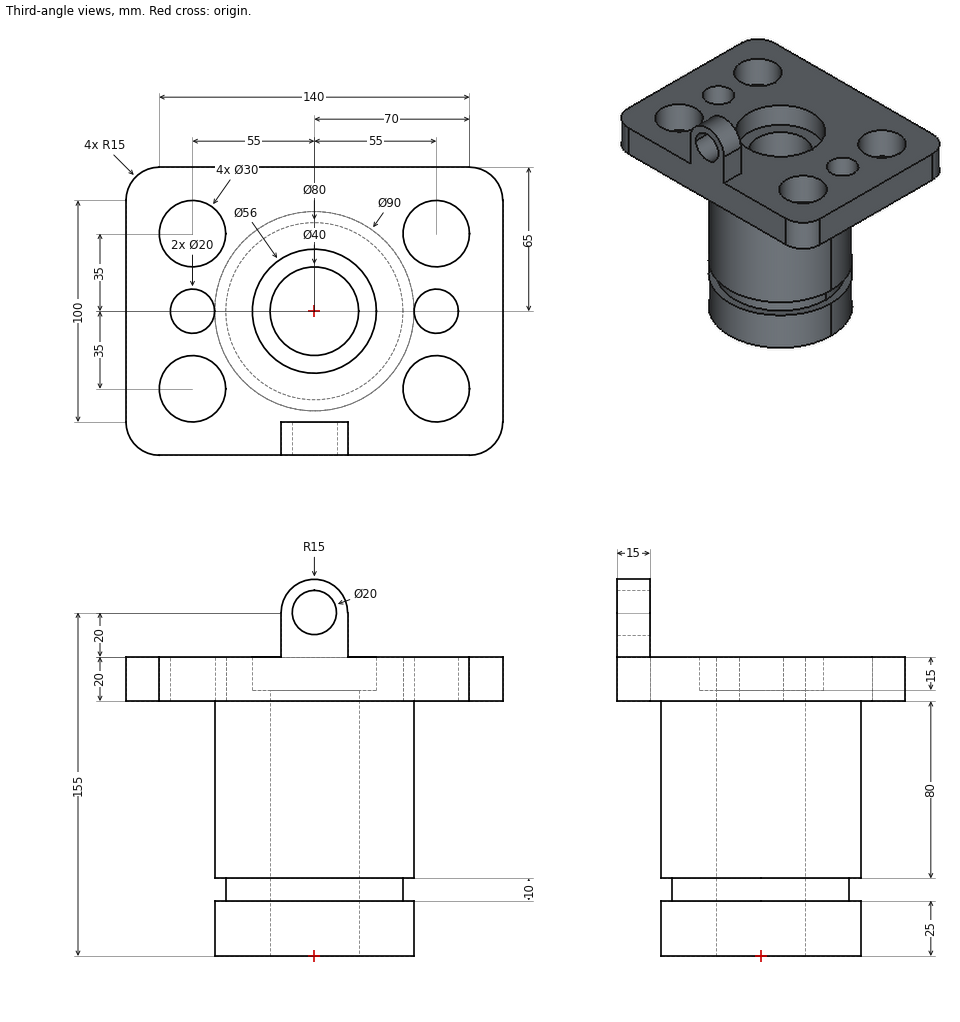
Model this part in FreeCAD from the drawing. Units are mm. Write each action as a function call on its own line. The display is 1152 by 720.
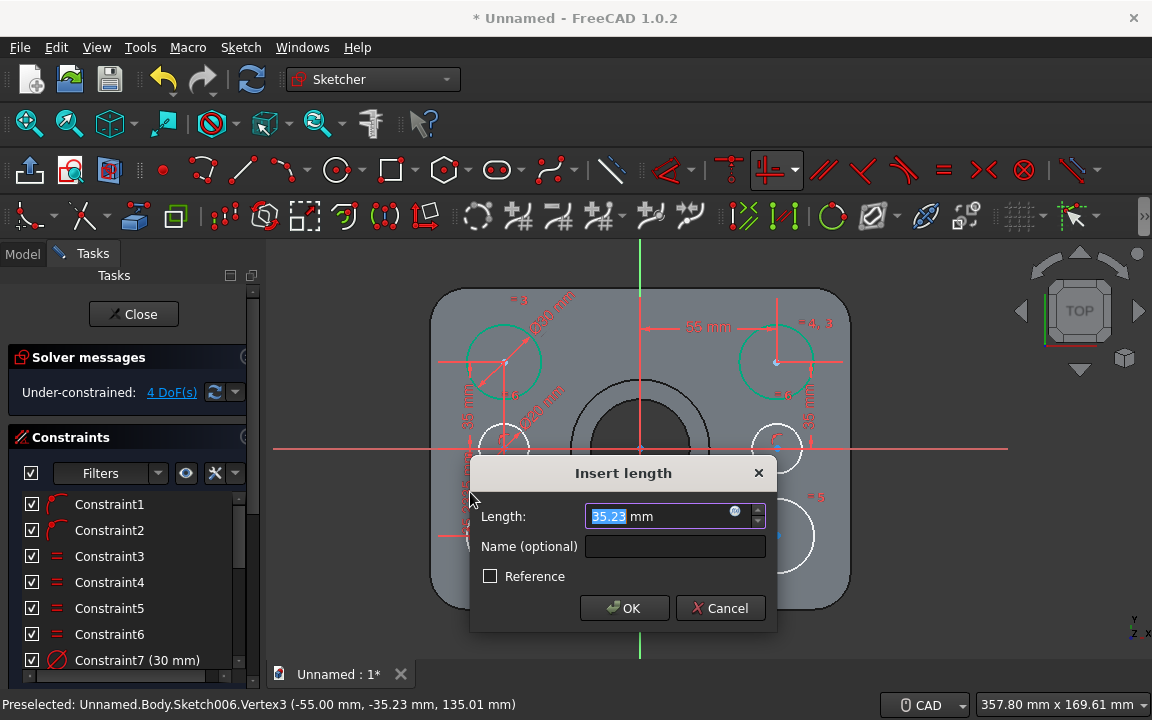
text(35)
key(Return)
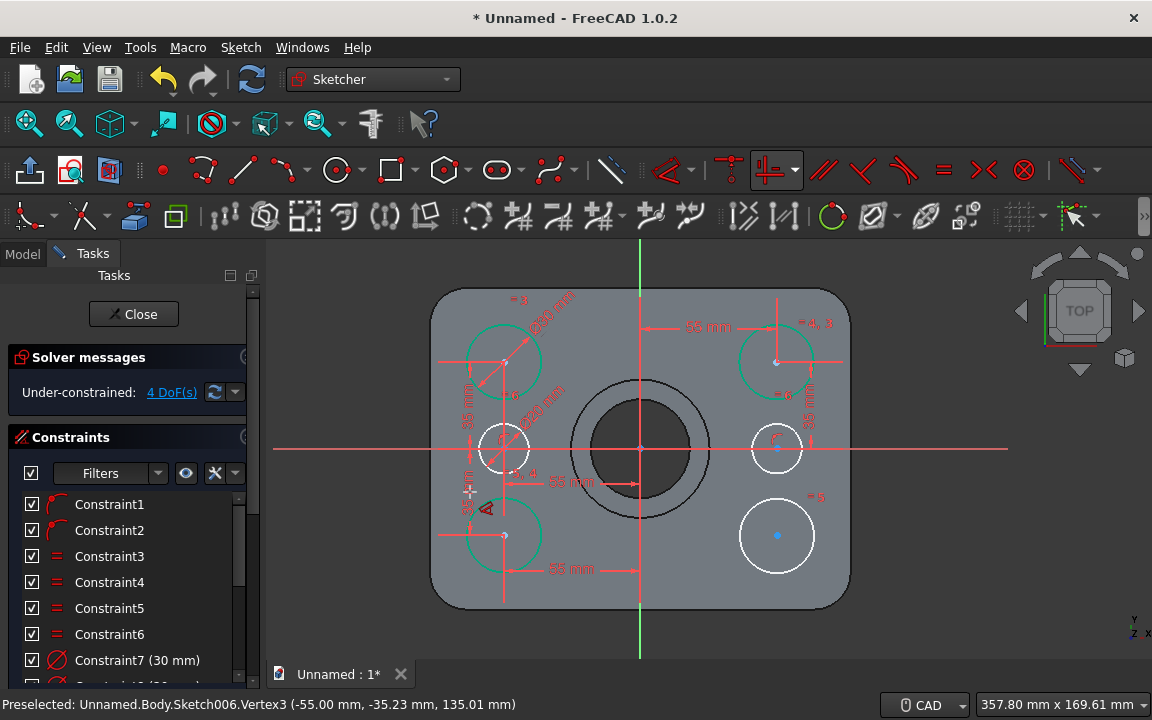
click(777, 536)
click(709, 570)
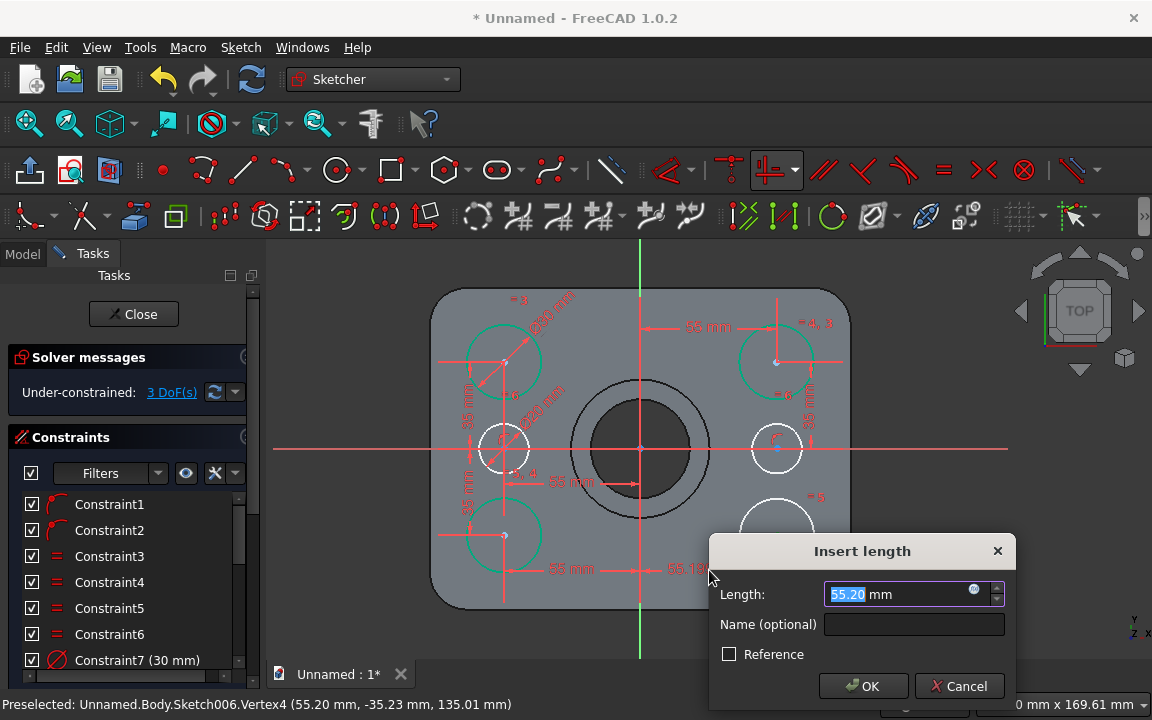
text(55)
key(Return)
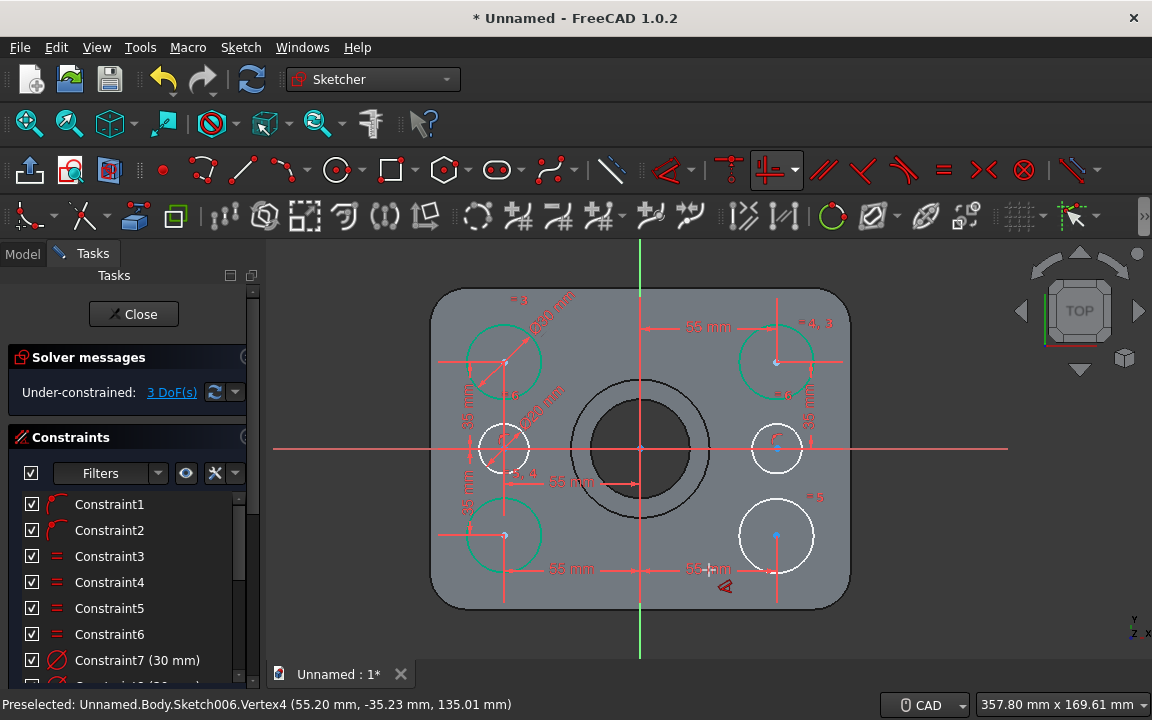
click(777, 536)
click(811, 492)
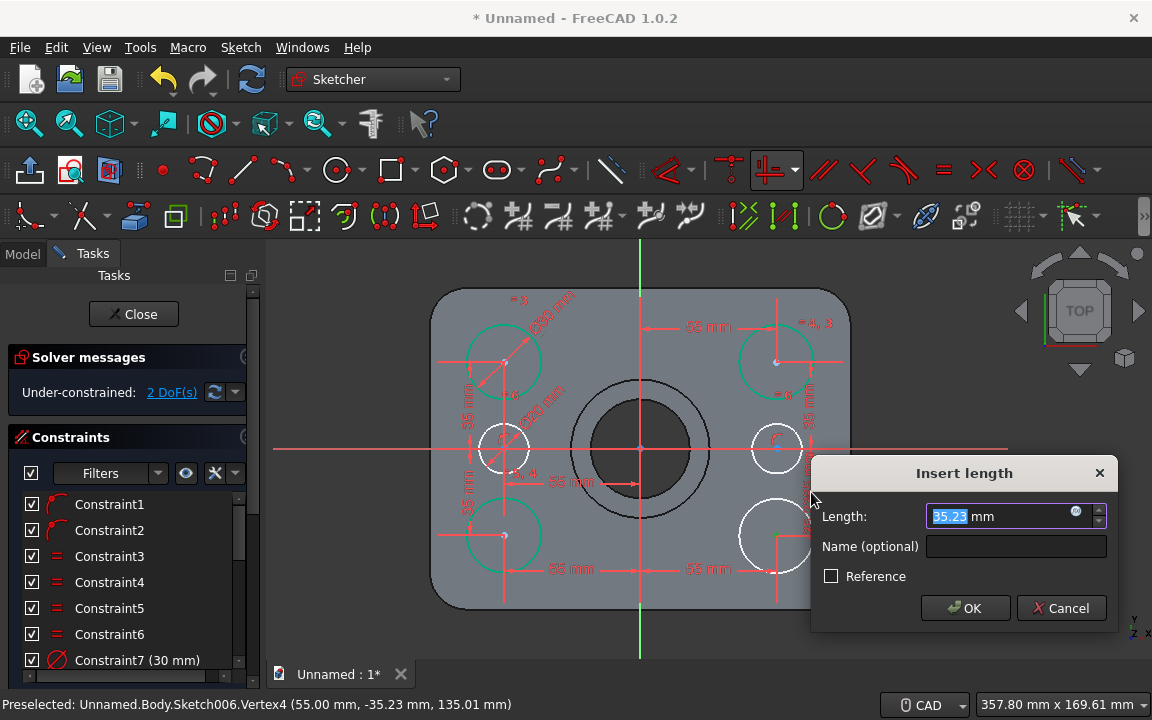
text(35)
key(Return)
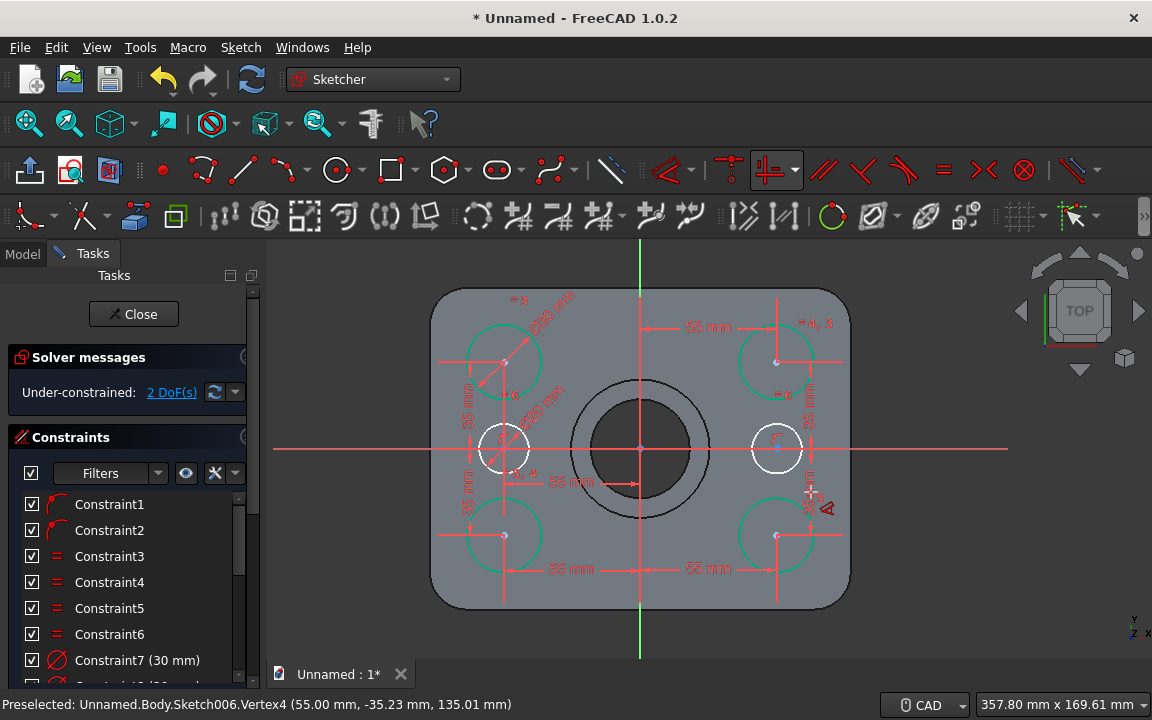
click(504, 449)
click(620, 415)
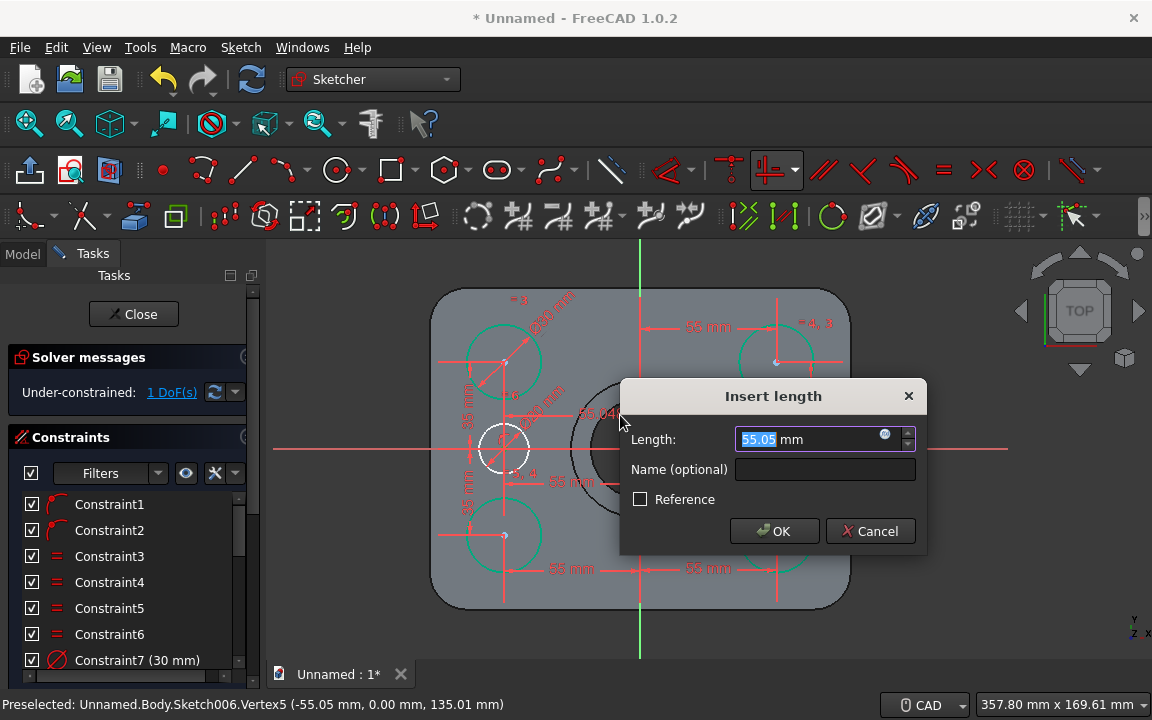
text(55)
key(Return)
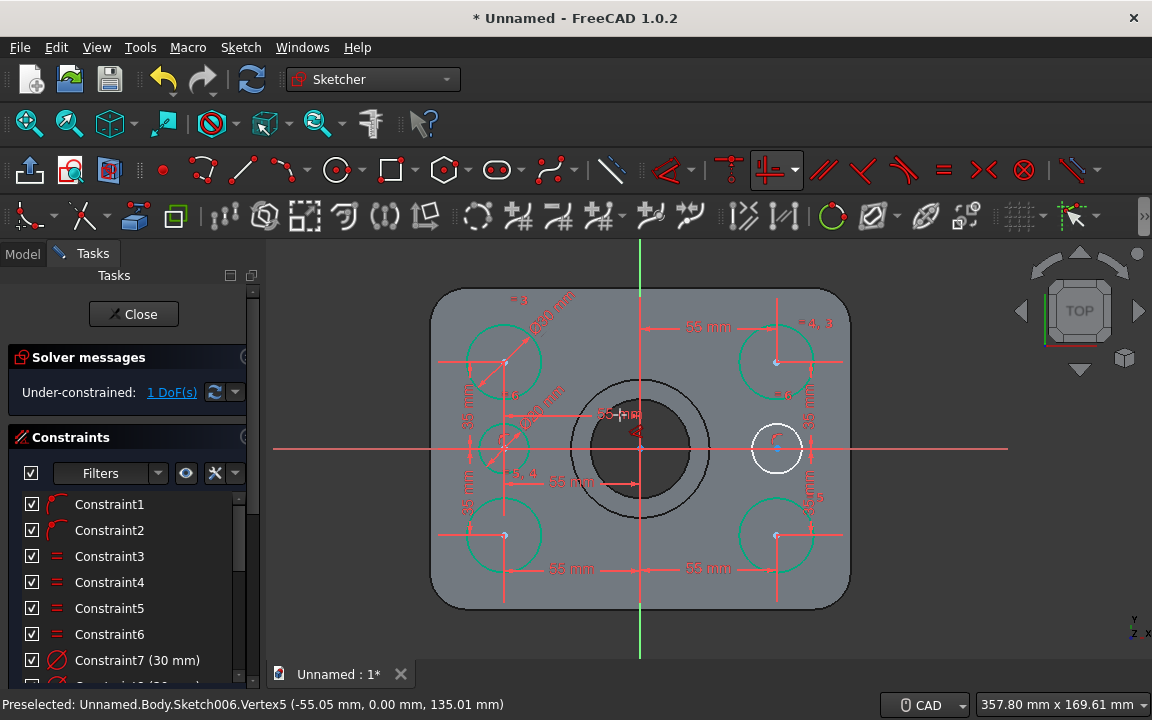
click(777, 449)
click(709, 483)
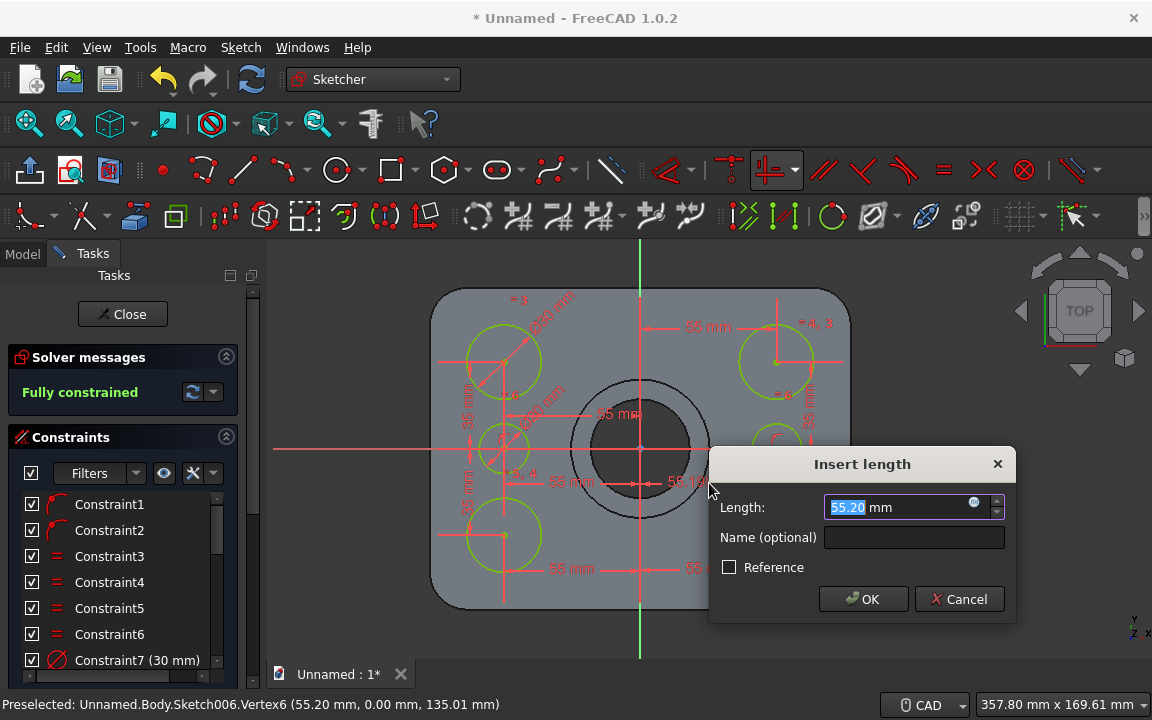
text(55)
key(Return)
key(Escape)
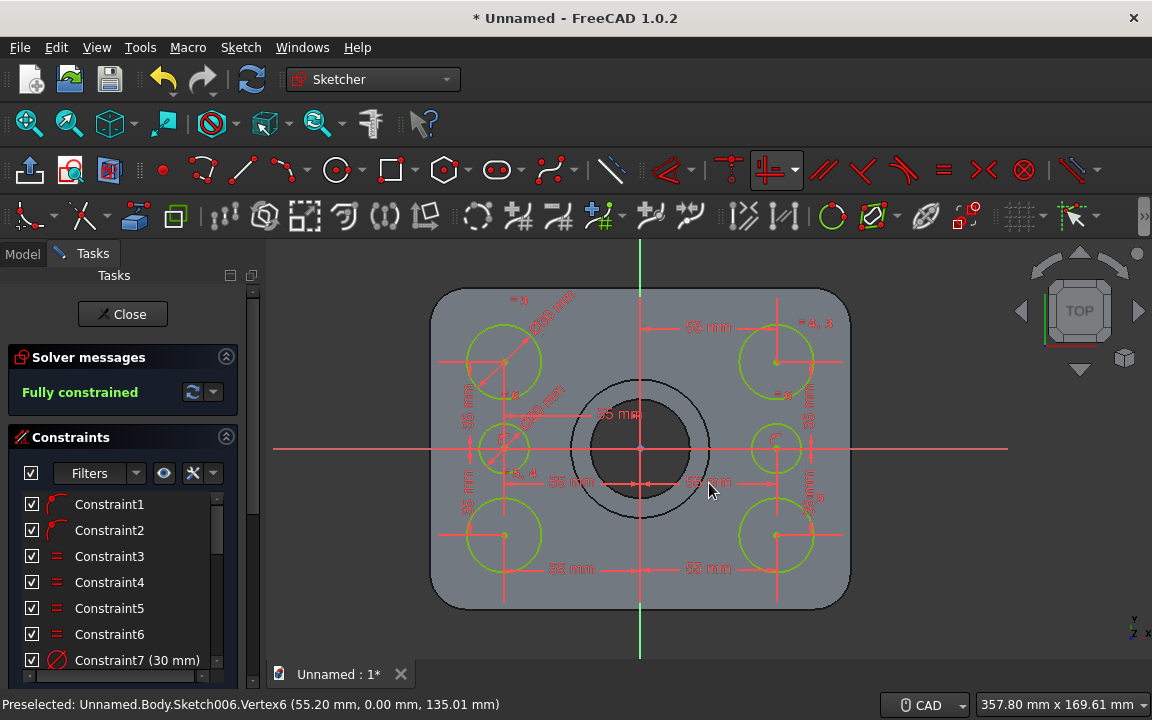
click(123, 314)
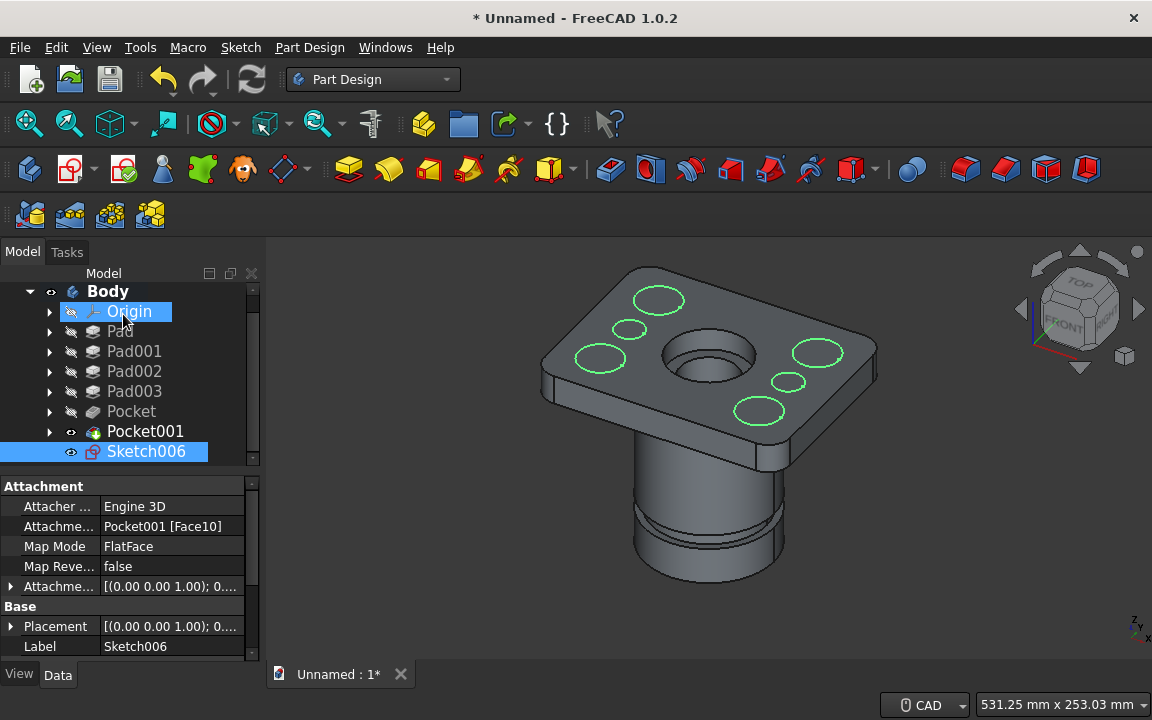
click(612, 170)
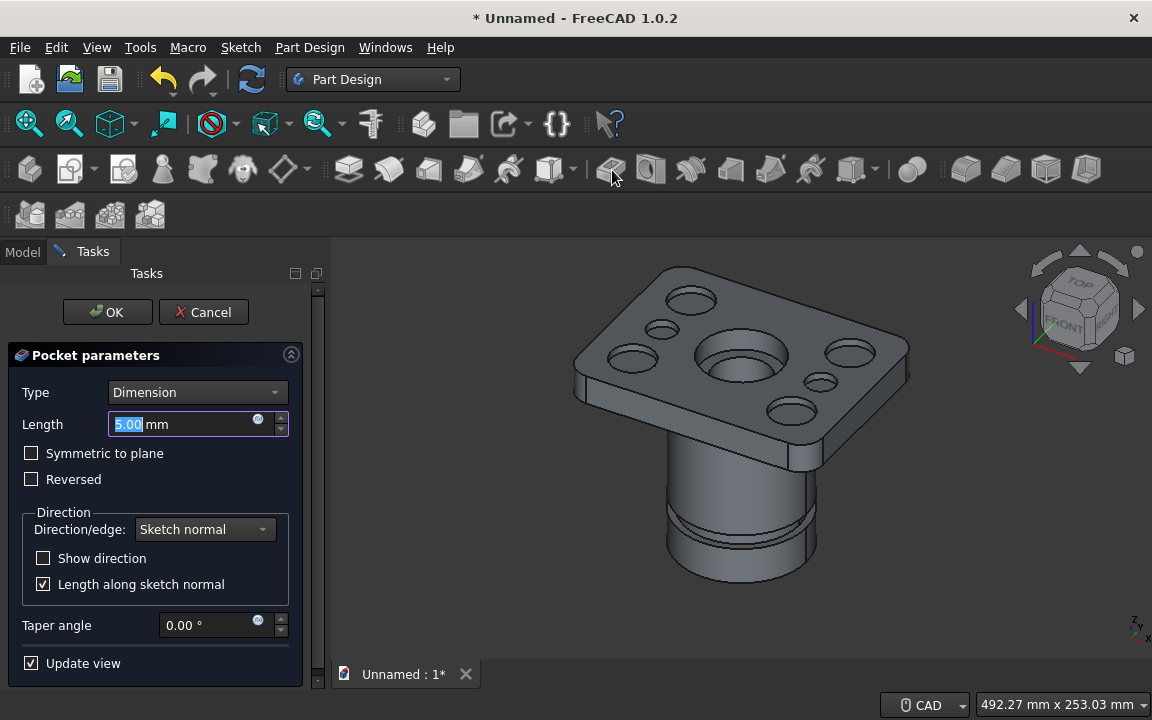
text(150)
key(Tab)